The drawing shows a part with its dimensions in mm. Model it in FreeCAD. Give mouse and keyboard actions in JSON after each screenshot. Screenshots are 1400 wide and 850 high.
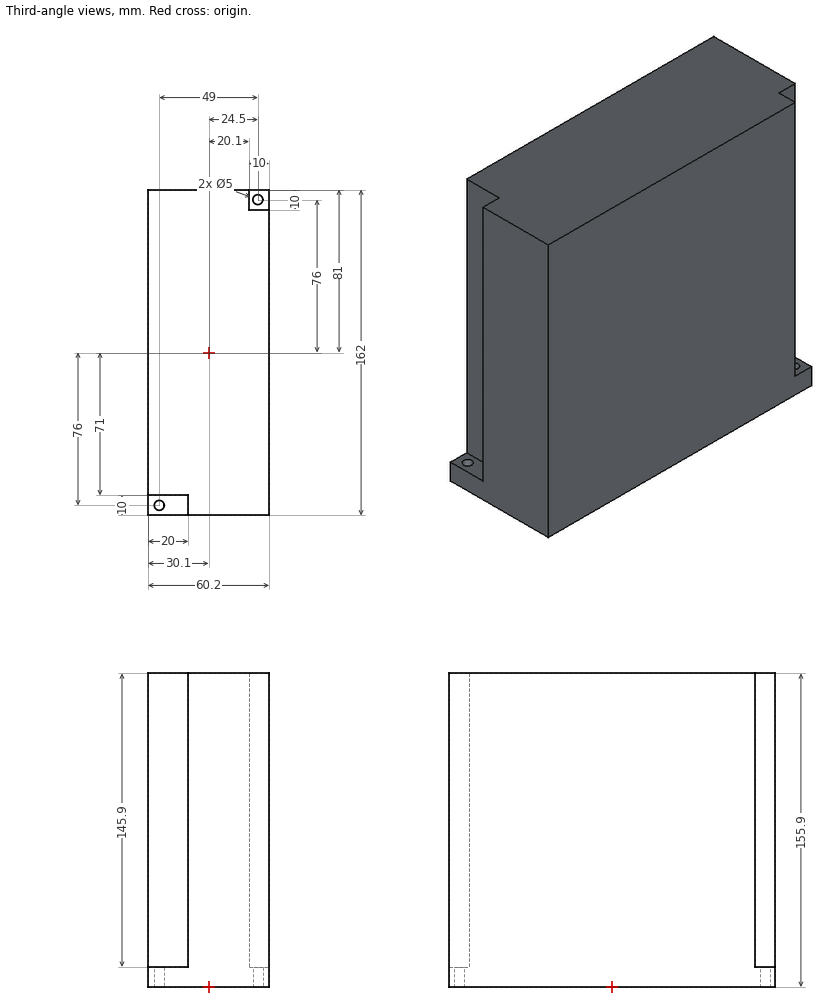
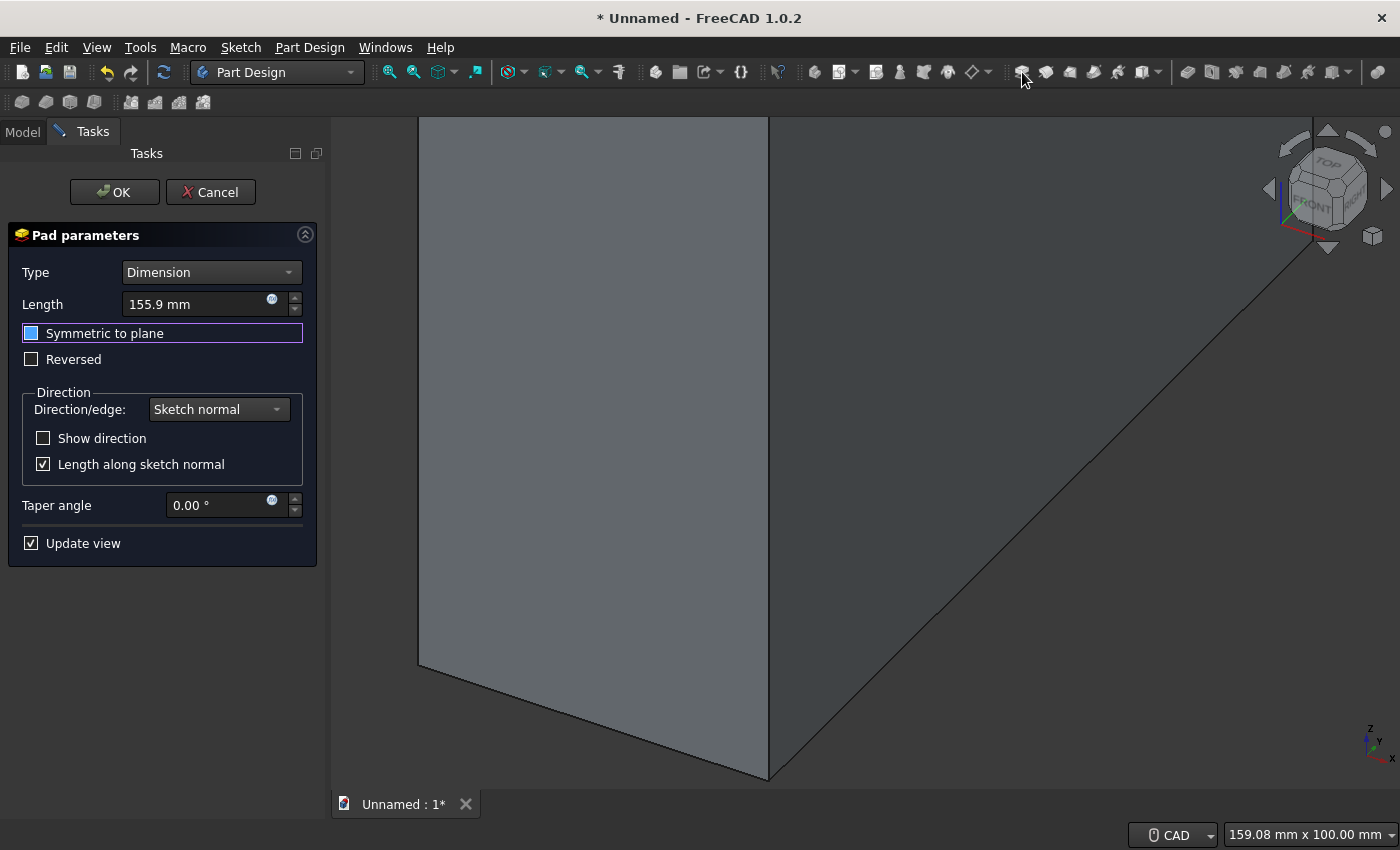
{"action": "left_click", "coordinate": [115, 192]}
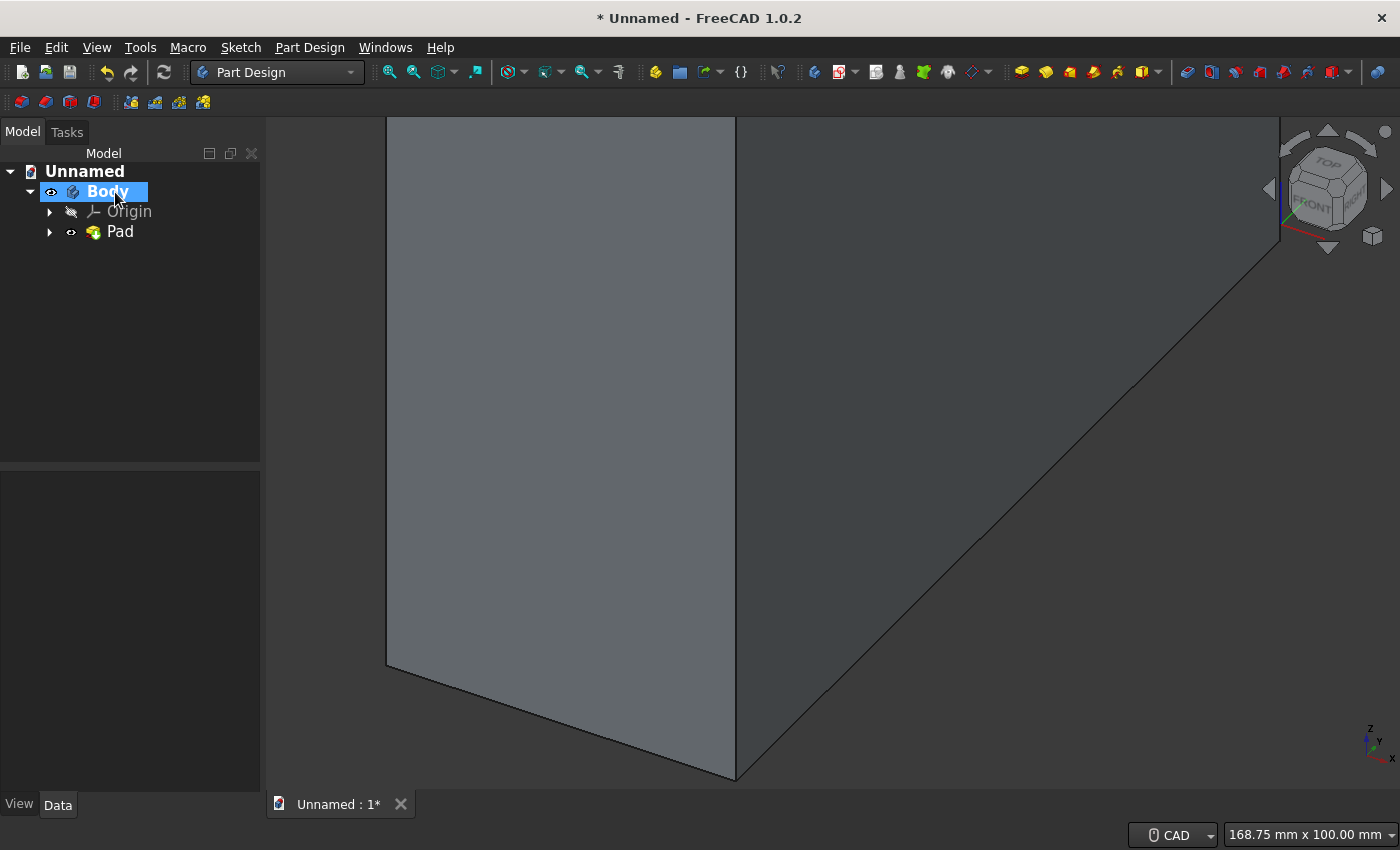
{"action": "key", "text": "v f"}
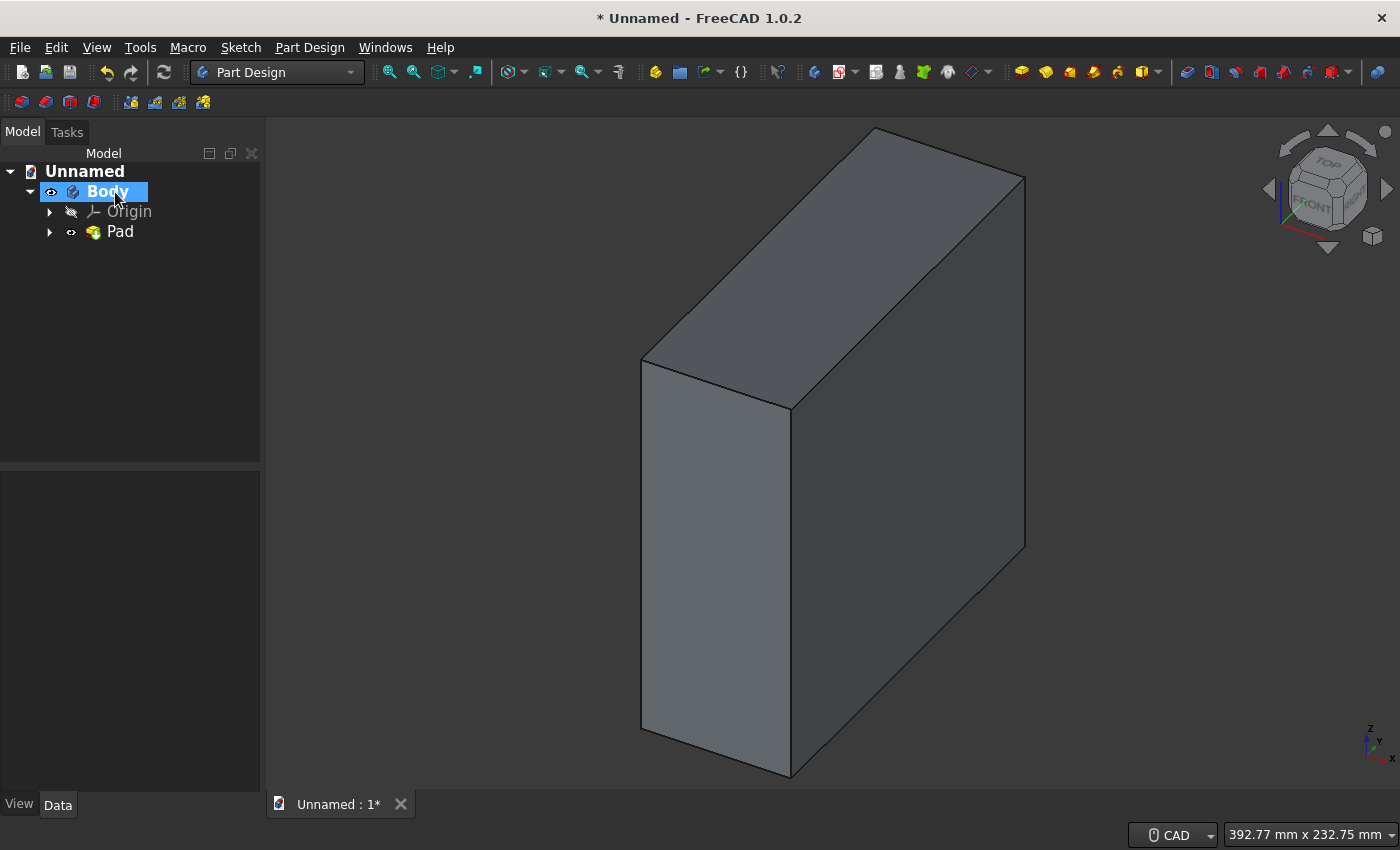
{"action": "left_click", "coordinate": [900, 201]}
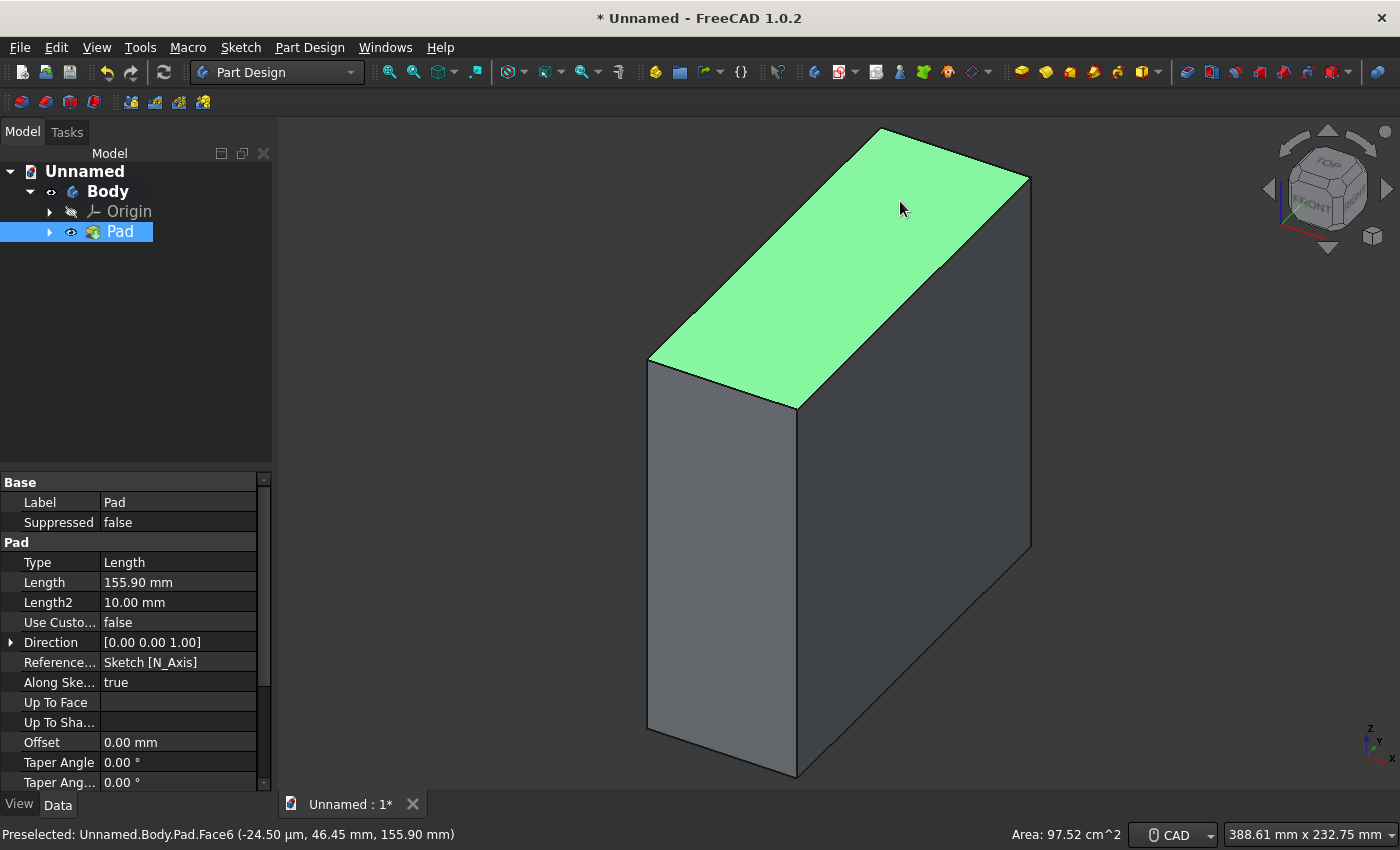
{"action": "left_click", "coordinate": [840, 72]}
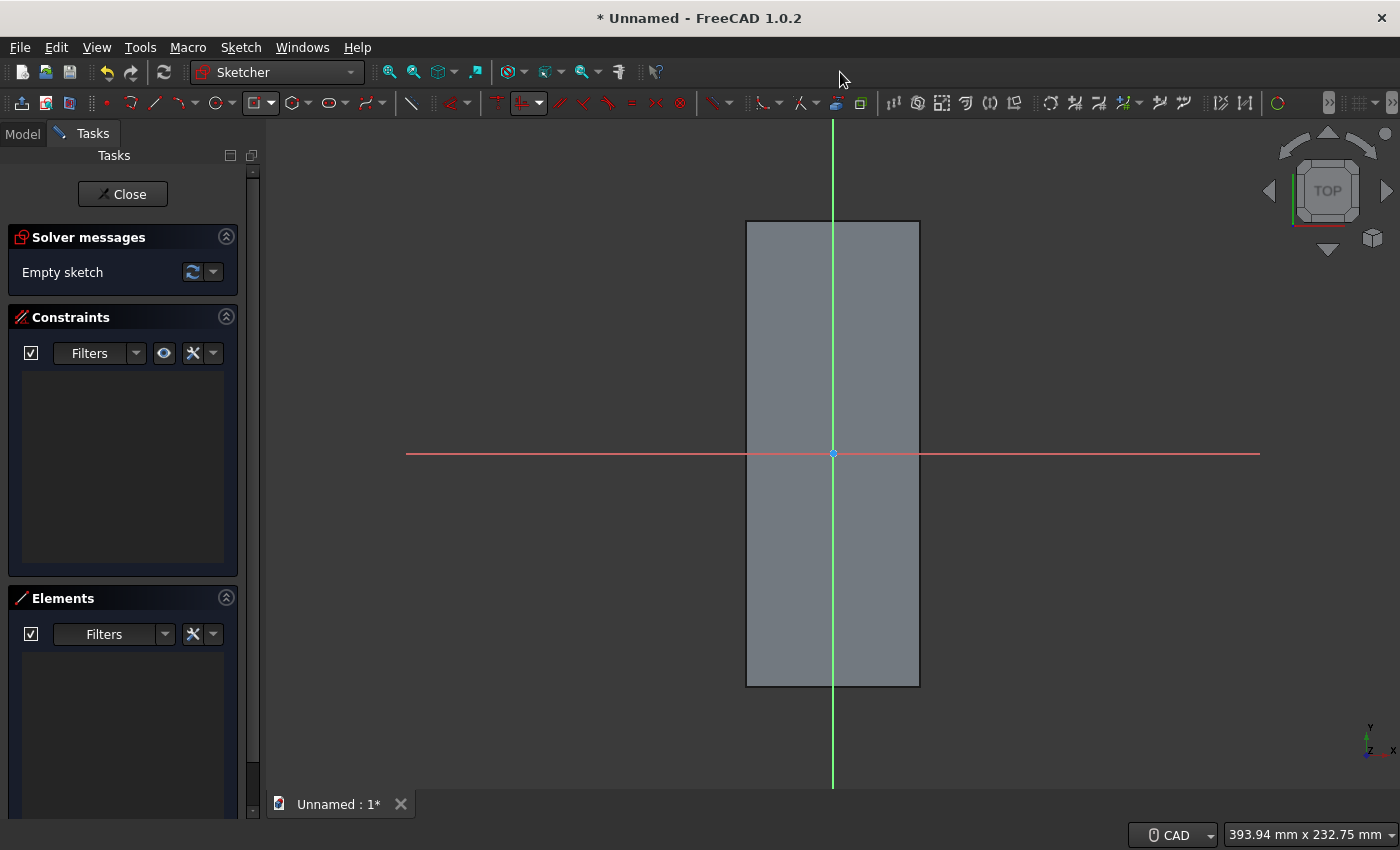
{"action": "left_click", "coordinate": [274, 104]}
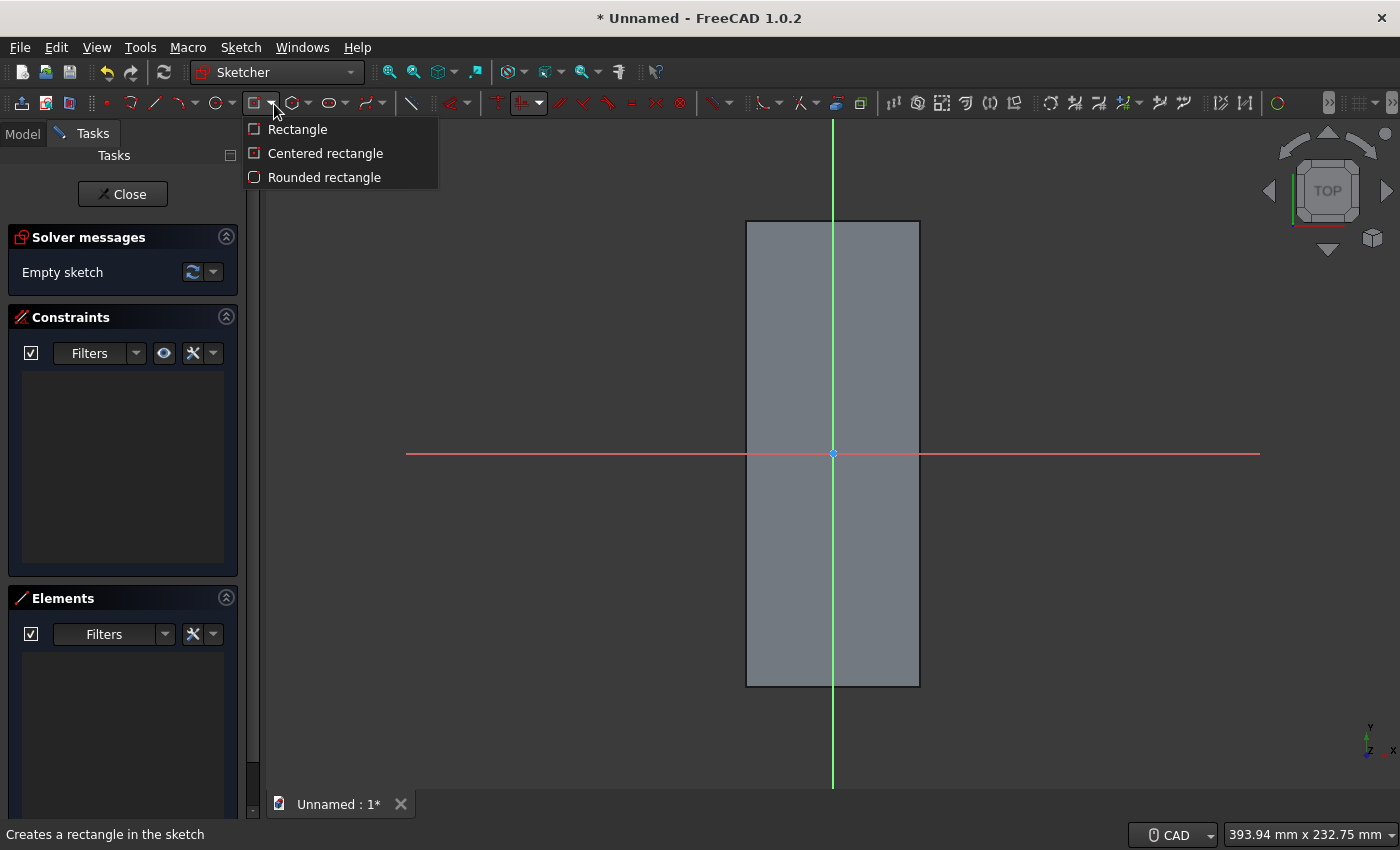
{"action": "left_click", "coordinate": [340, 129]}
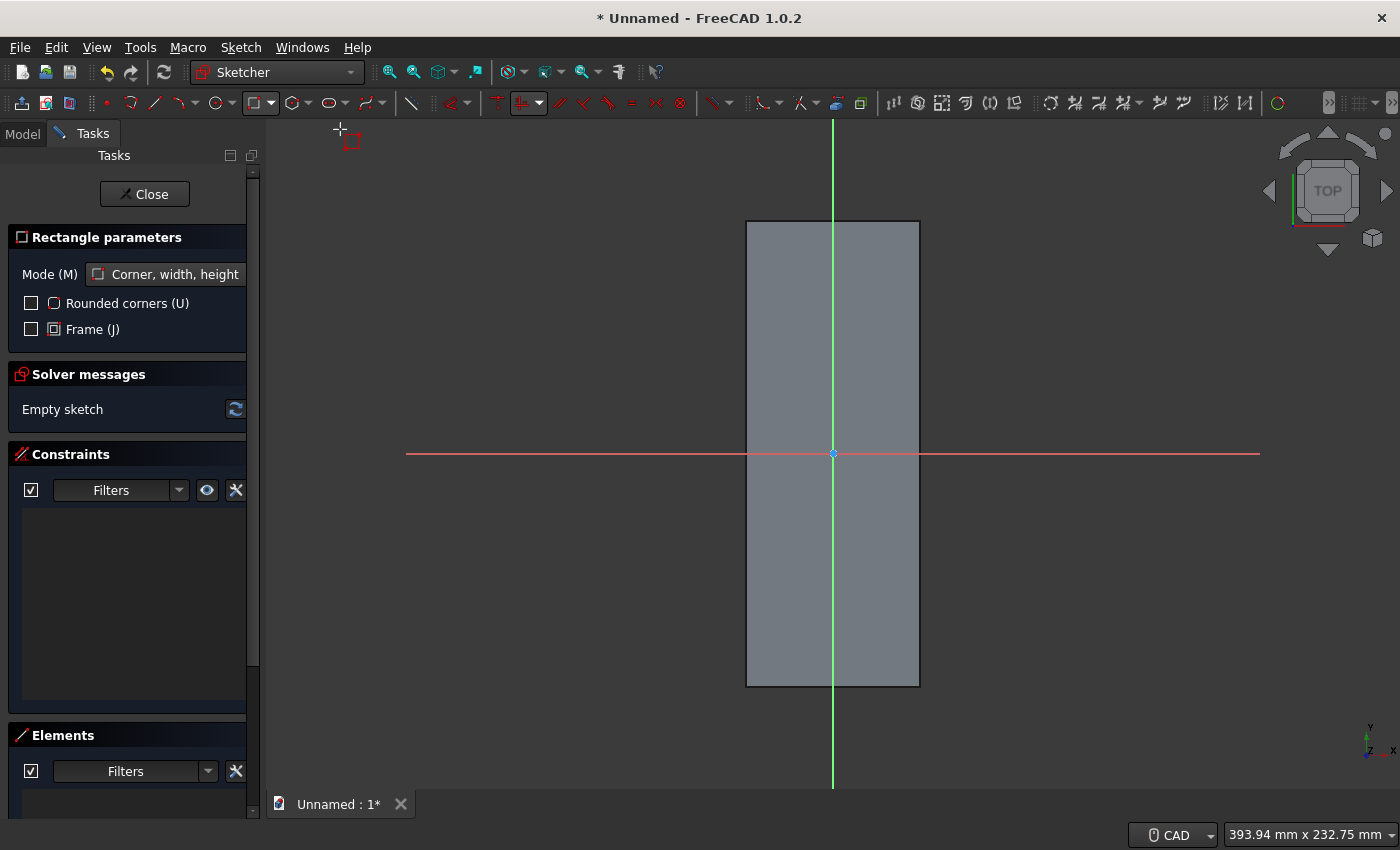
{"action": "left_click", "coordinate": [746, 658]}
{"action": "left_click", "coordinate": [804, 687]}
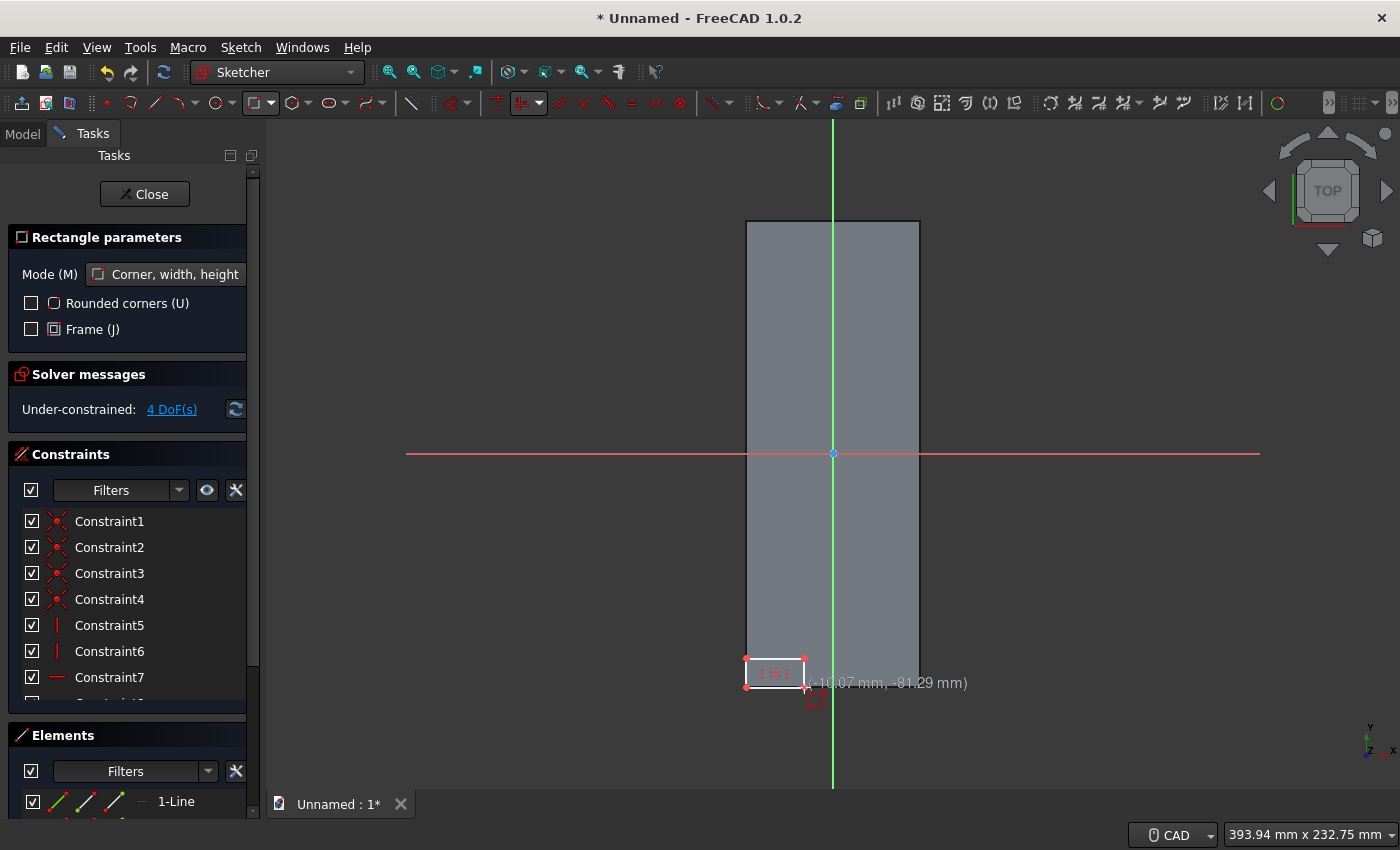
{"action": "left_click", "coordinate": [891, 221]}
{"action": "left_click", "coordinate": [920, 250]}
{"action": "key", "text": "Escape"}